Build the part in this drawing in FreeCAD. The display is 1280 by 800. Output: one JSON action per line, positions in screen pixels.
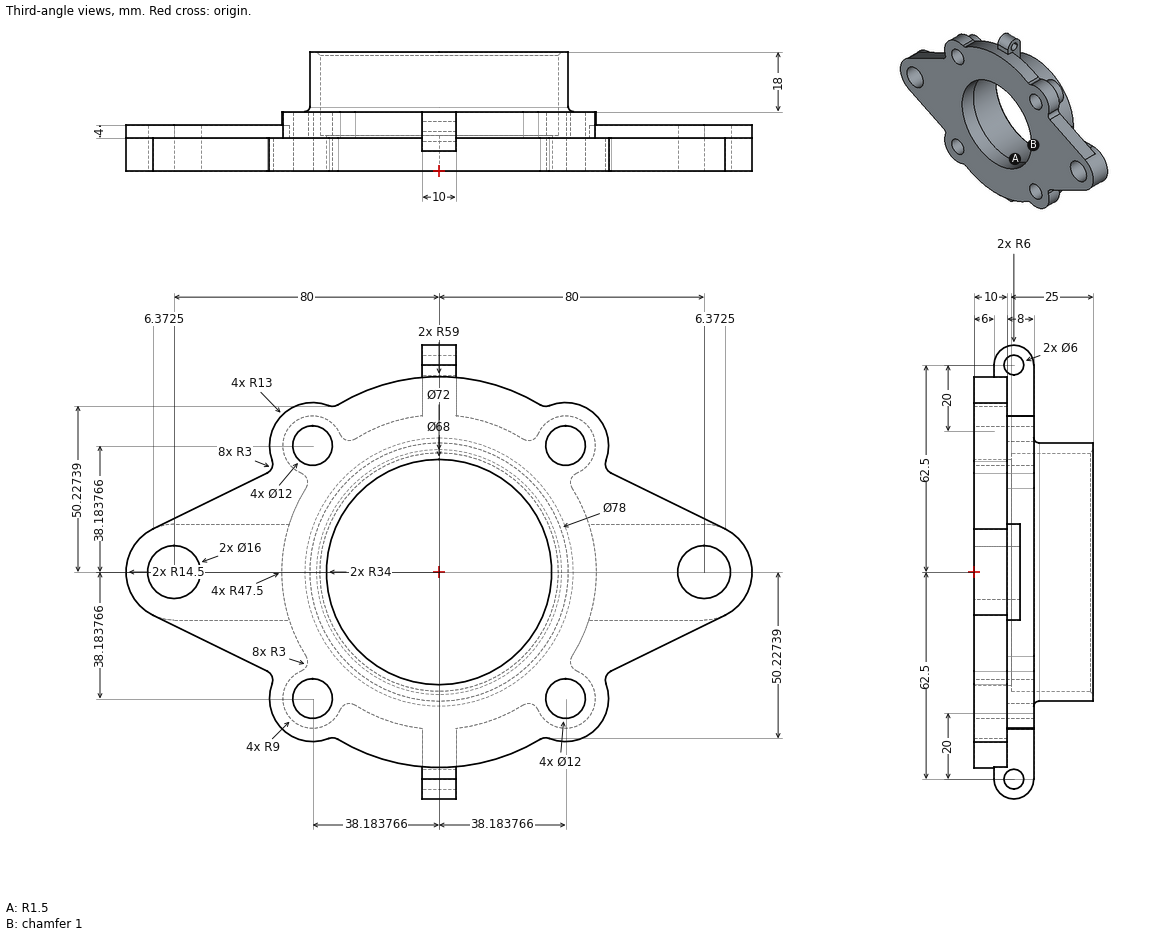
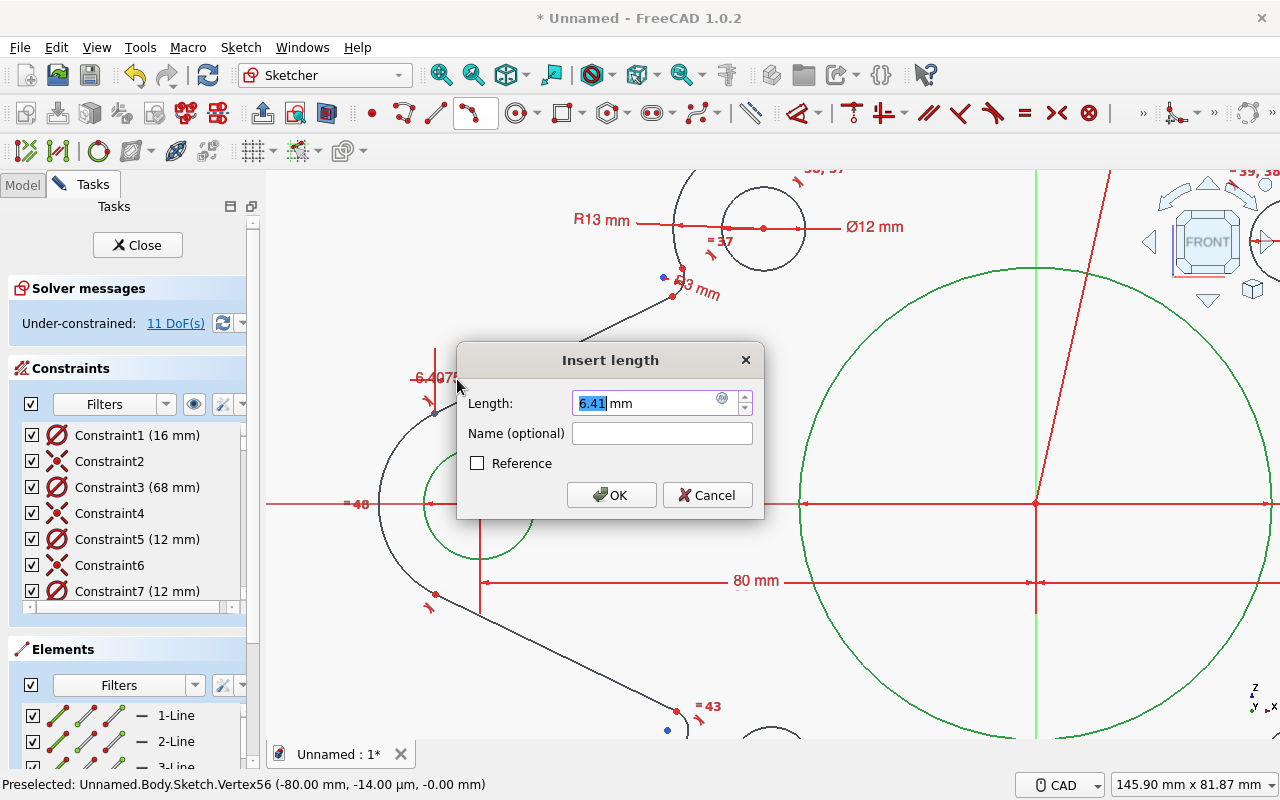
{"action": "type", "text": "6.3725"}
{"action": "key", "text": "Return"}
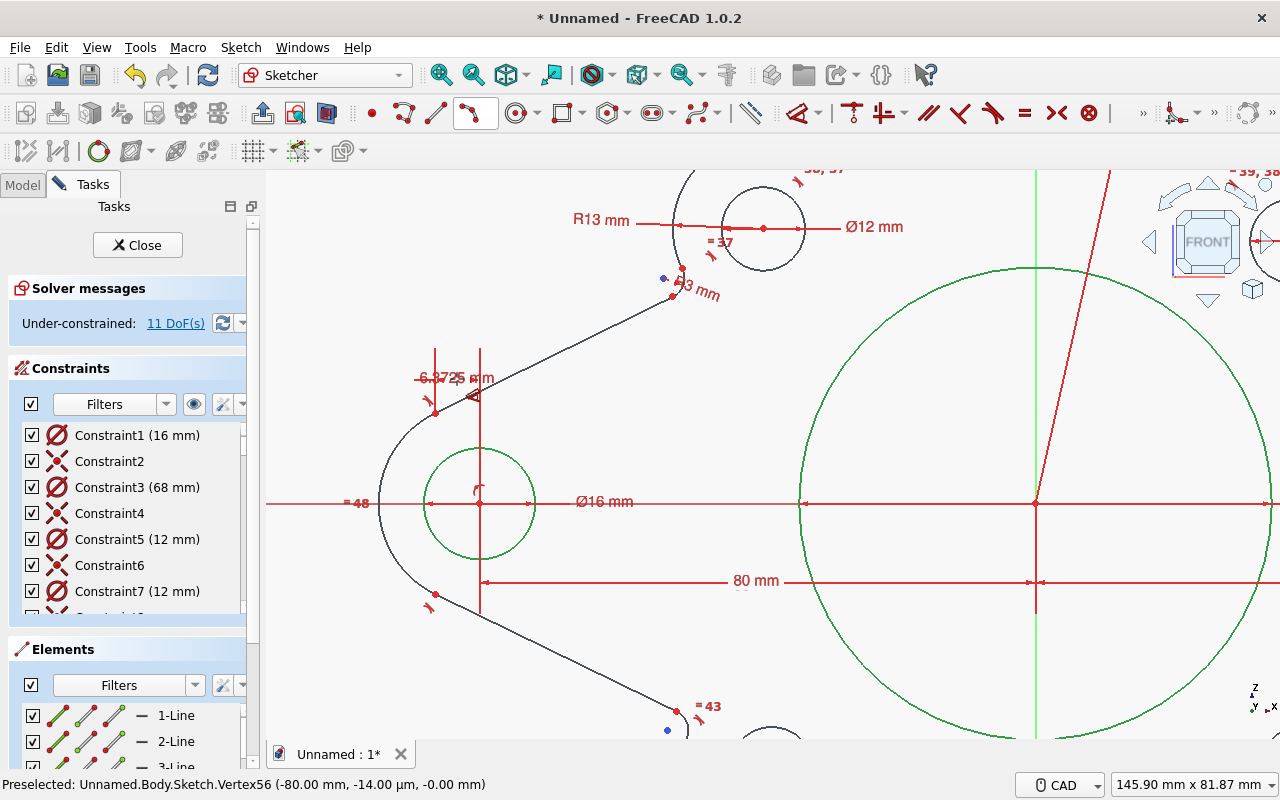
{"action": "left_click", "coordinate": [436, 594]}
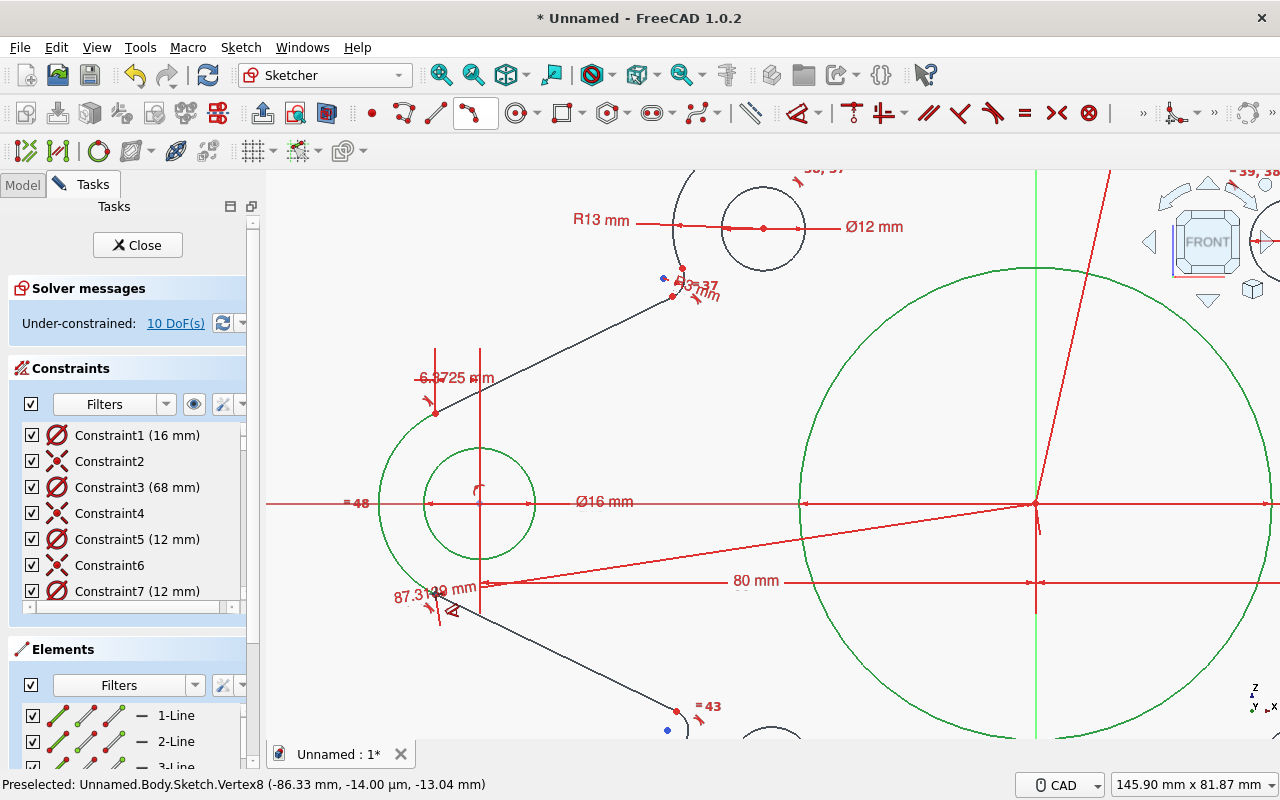
{"action": "left_click", "coordinate": [480, 504]}
{"action": "left_click", "coordinate": [458, 628]}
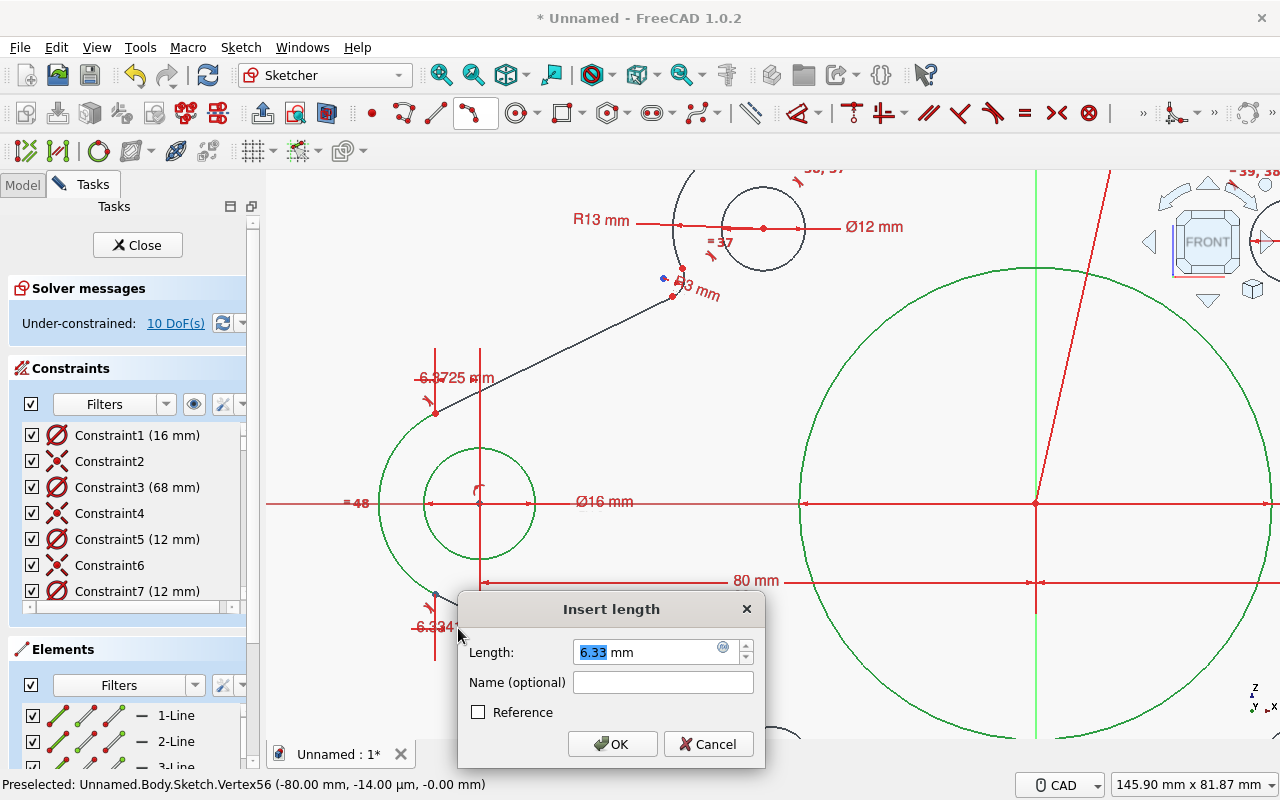
{"action": "type", "text": "6.3725"}
{"action": "key", "text": "Return"}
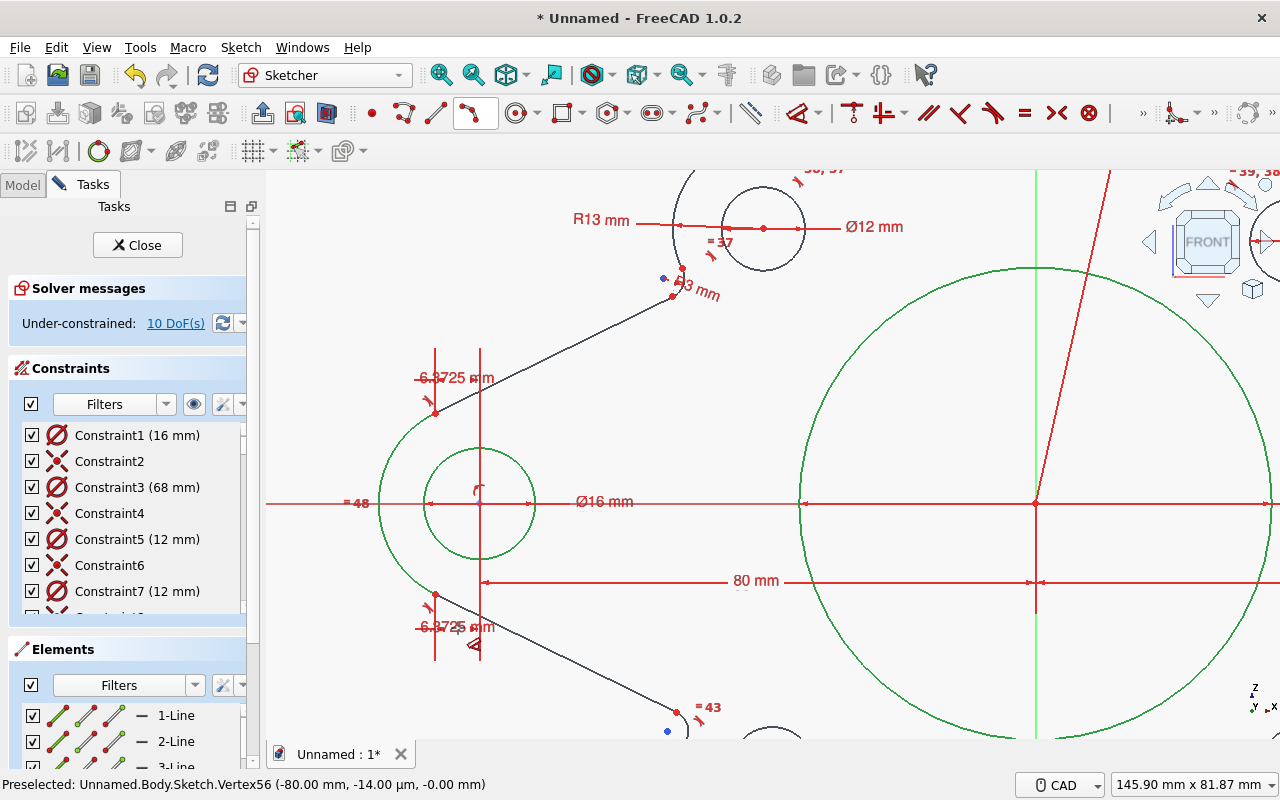
{"action": "scroll", "coordinate": [434, 414], "scroll_direction": "down", "scroll_amount": 4}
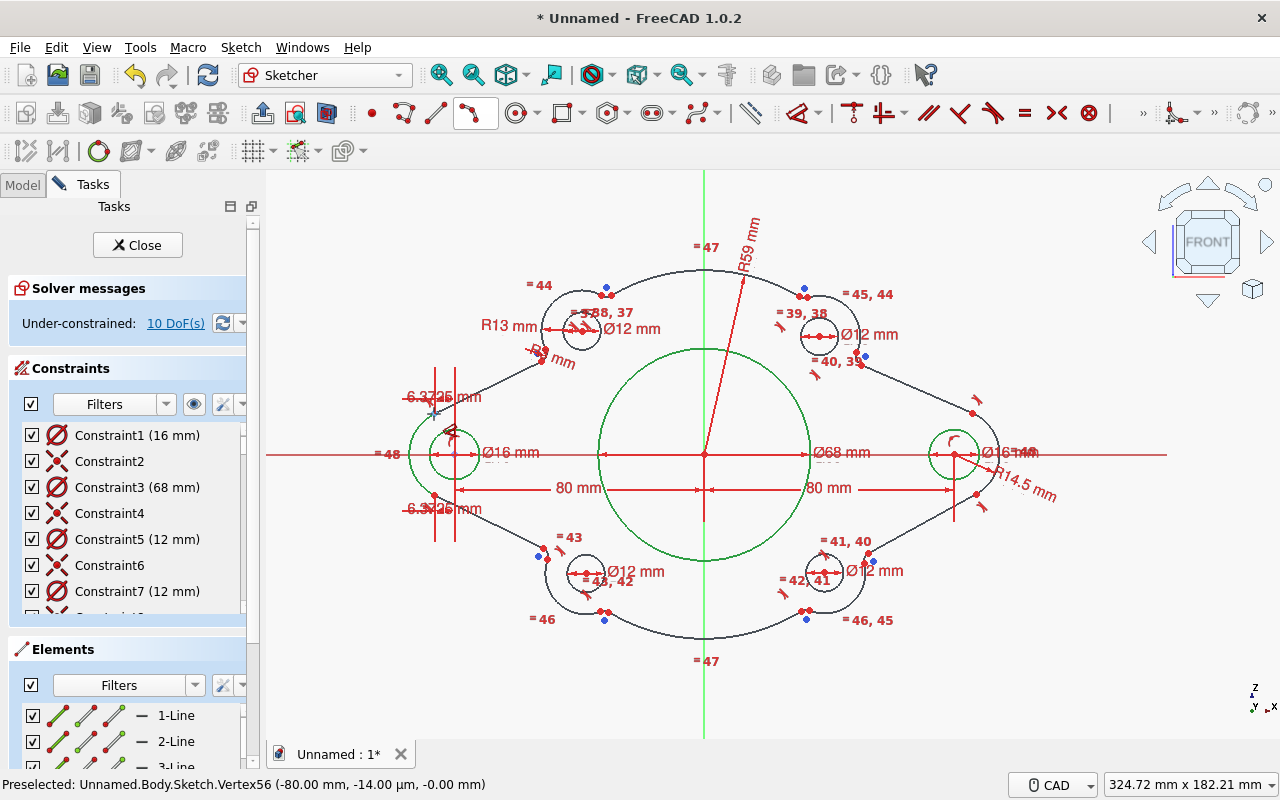
{"action": "scroll", "coordinate": [972, 413], "scroll_direction": "up", "scroll_amount": 4}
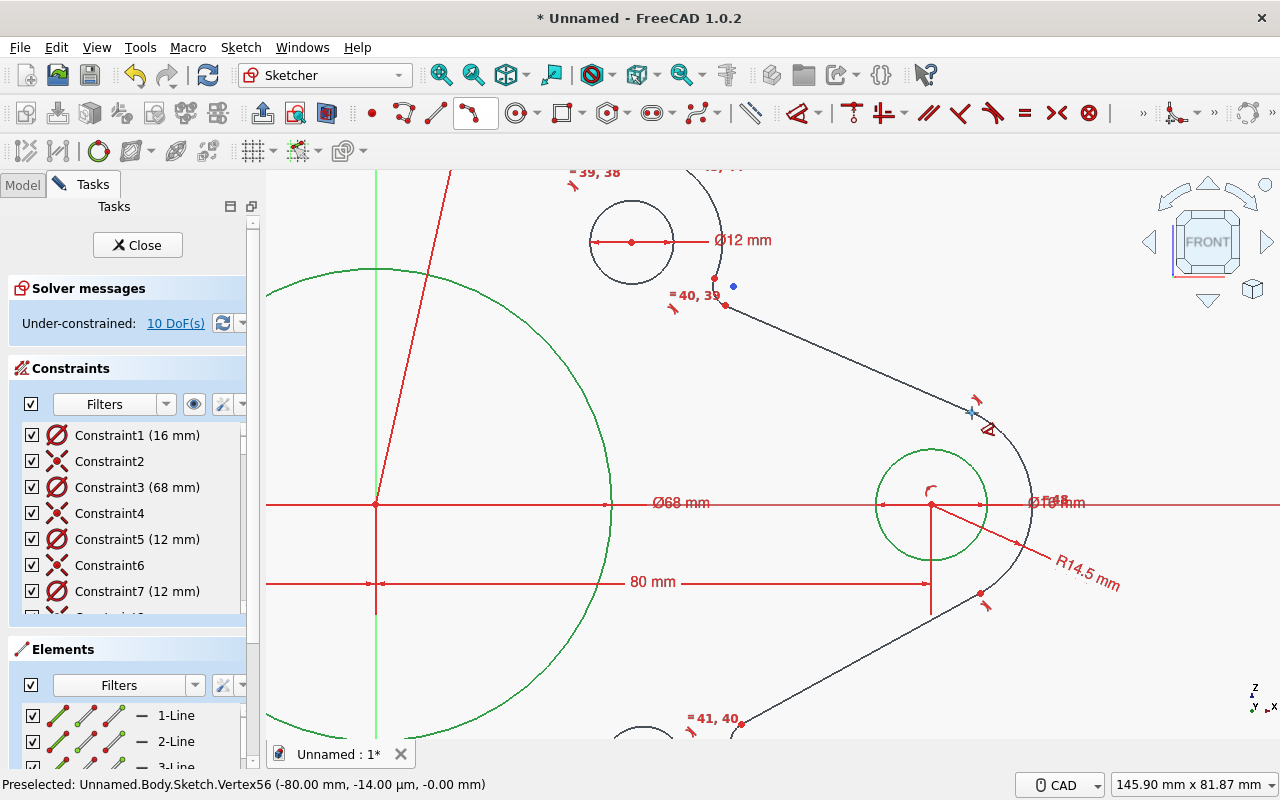
{"action": "left_click", "coordinate": [972, 412]}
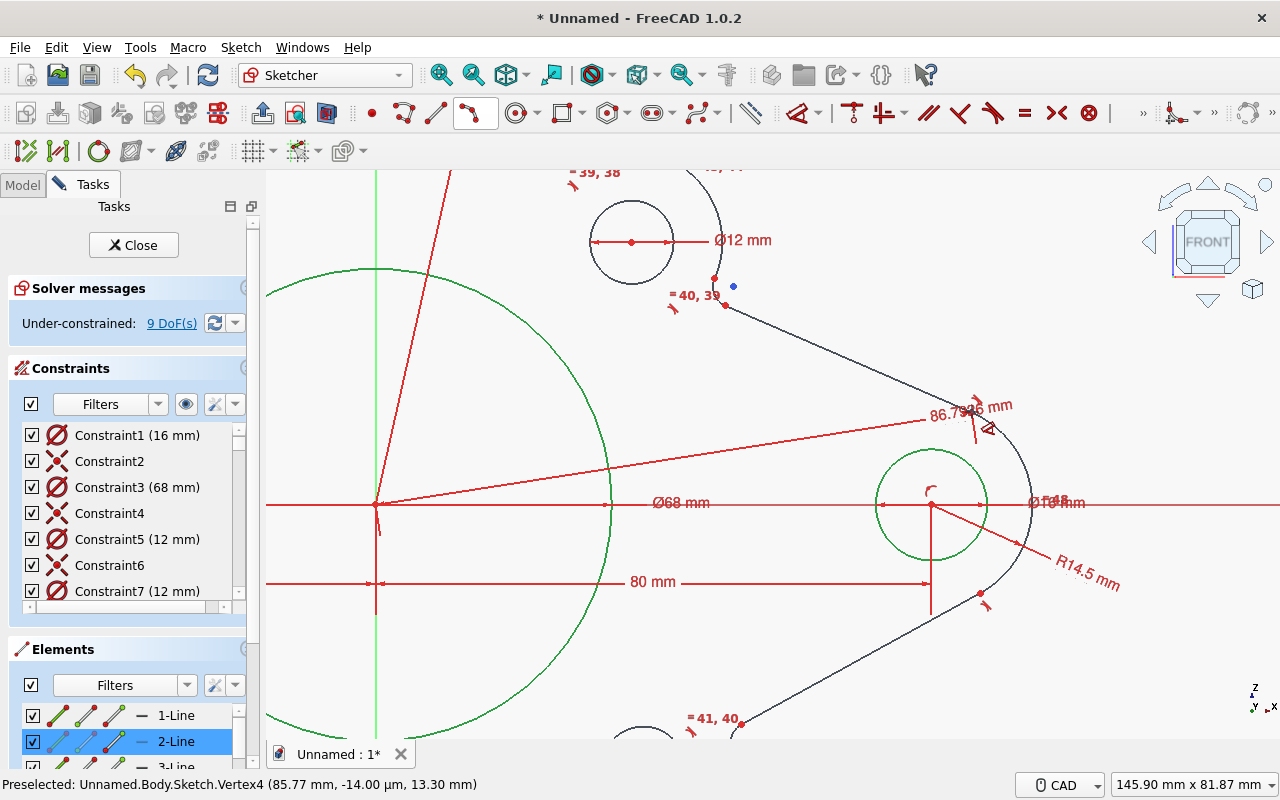
{"action": "left_click", "coordinate": [931, 505]}
{"action": "left_click", "coordinate": [952, 378]}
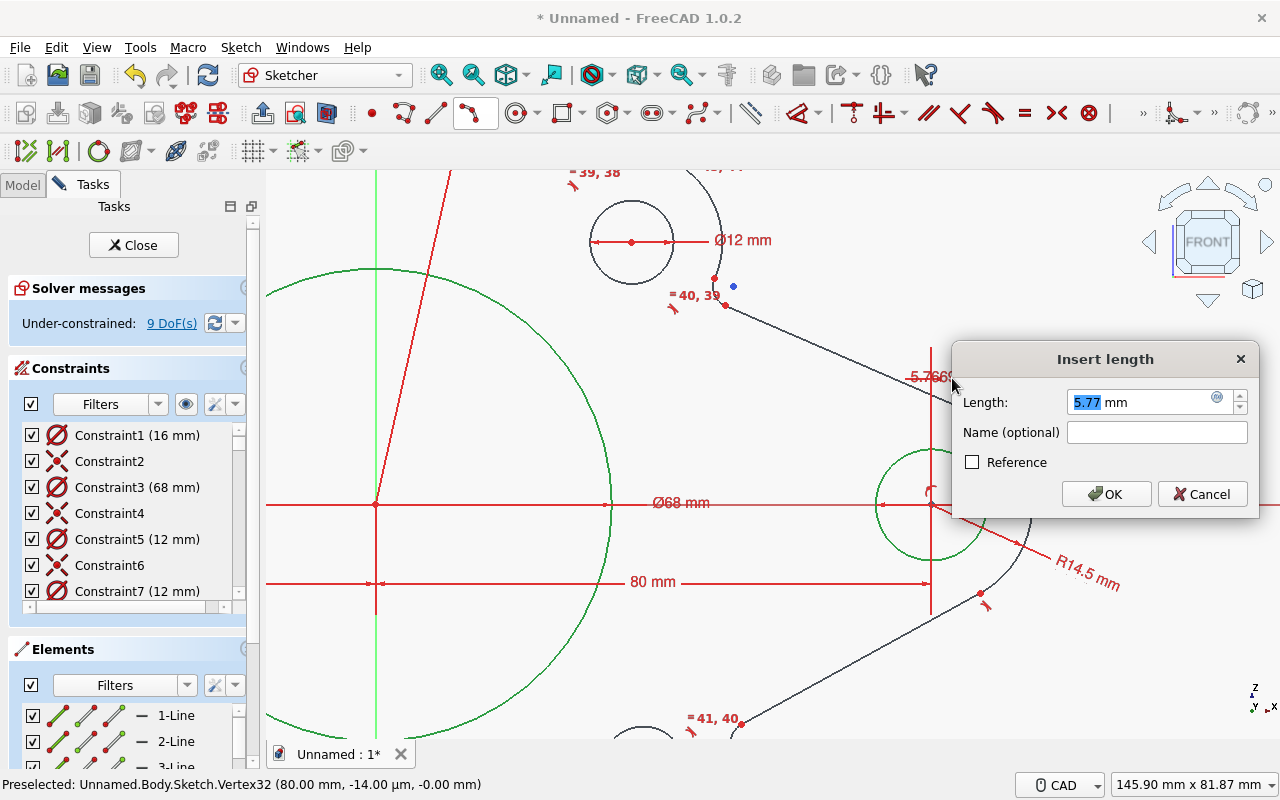
{"action": "type", "text": "6.3725"}
{"action": "key", "text": "Return"}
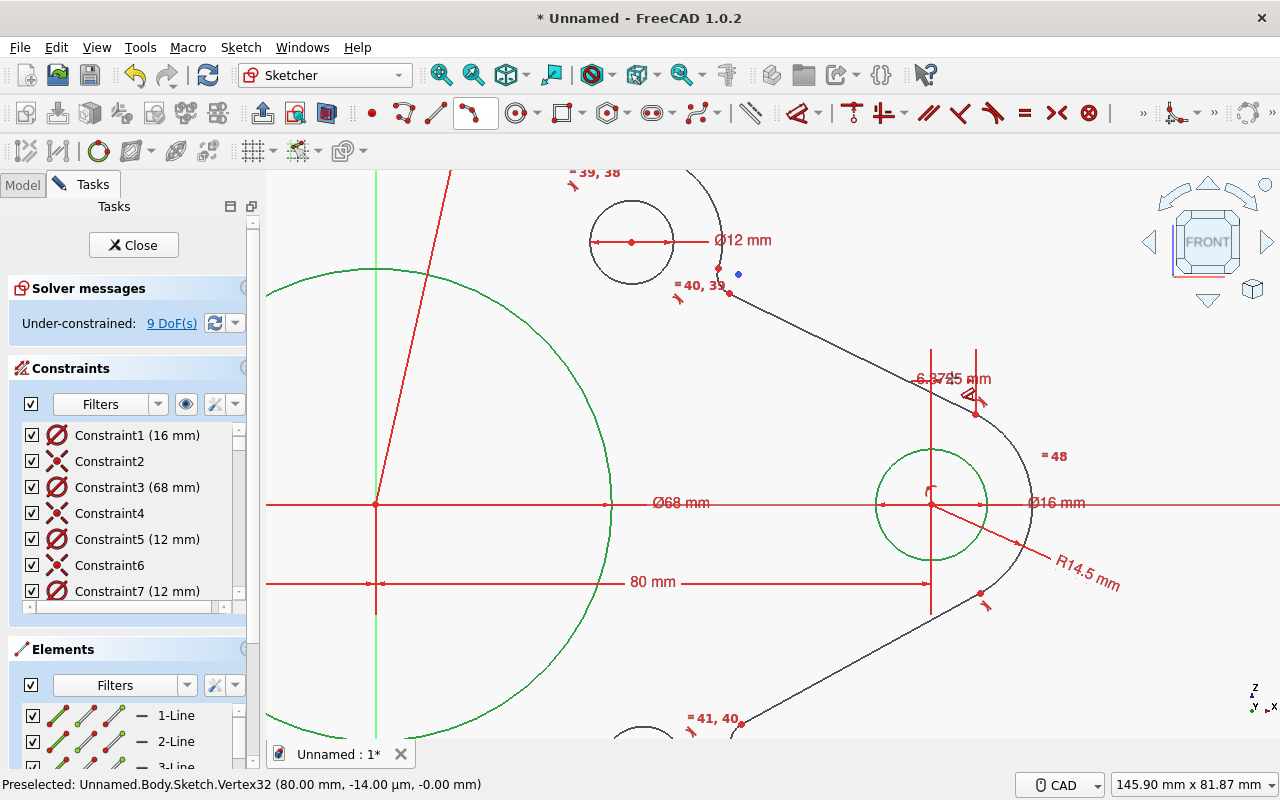
{"action": "left_click", "coordinate": [980, 593]}